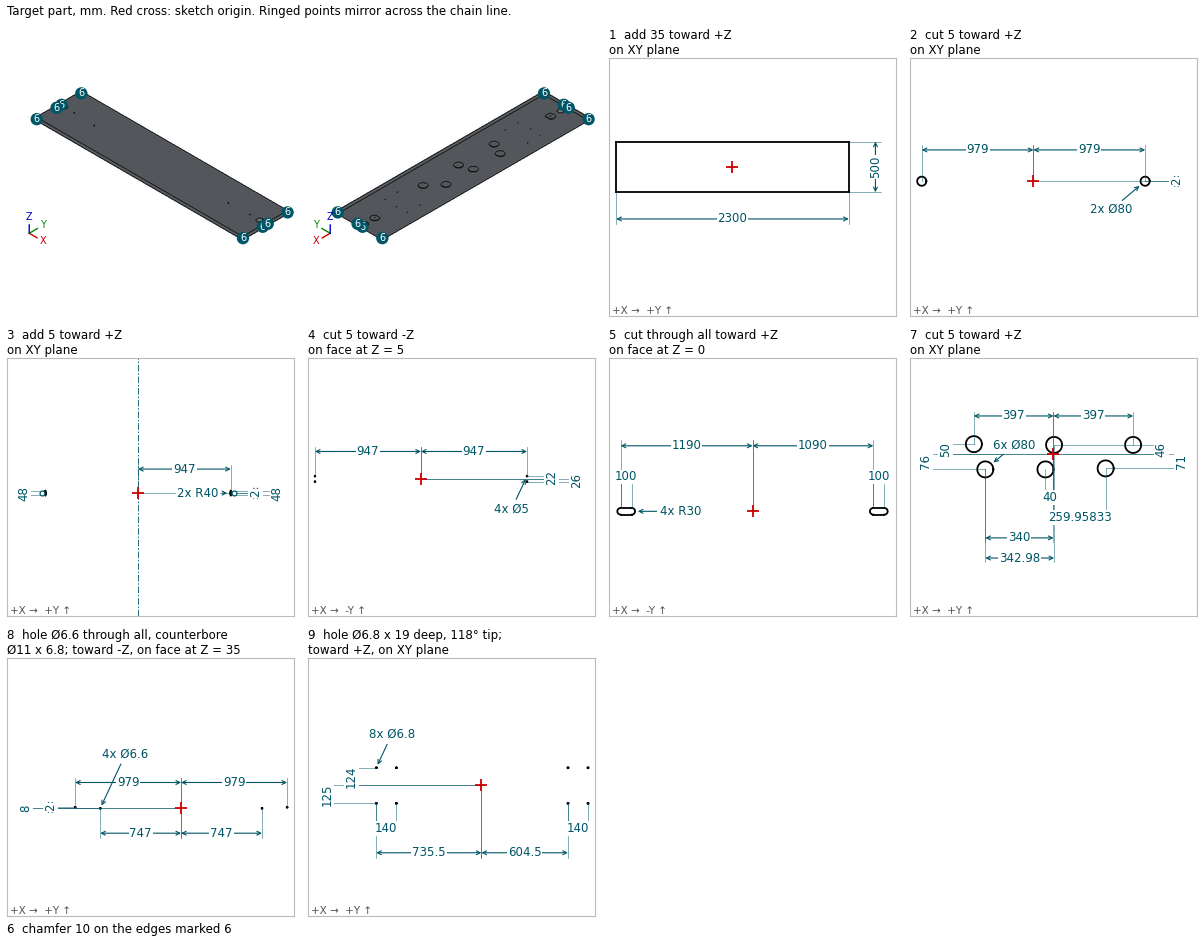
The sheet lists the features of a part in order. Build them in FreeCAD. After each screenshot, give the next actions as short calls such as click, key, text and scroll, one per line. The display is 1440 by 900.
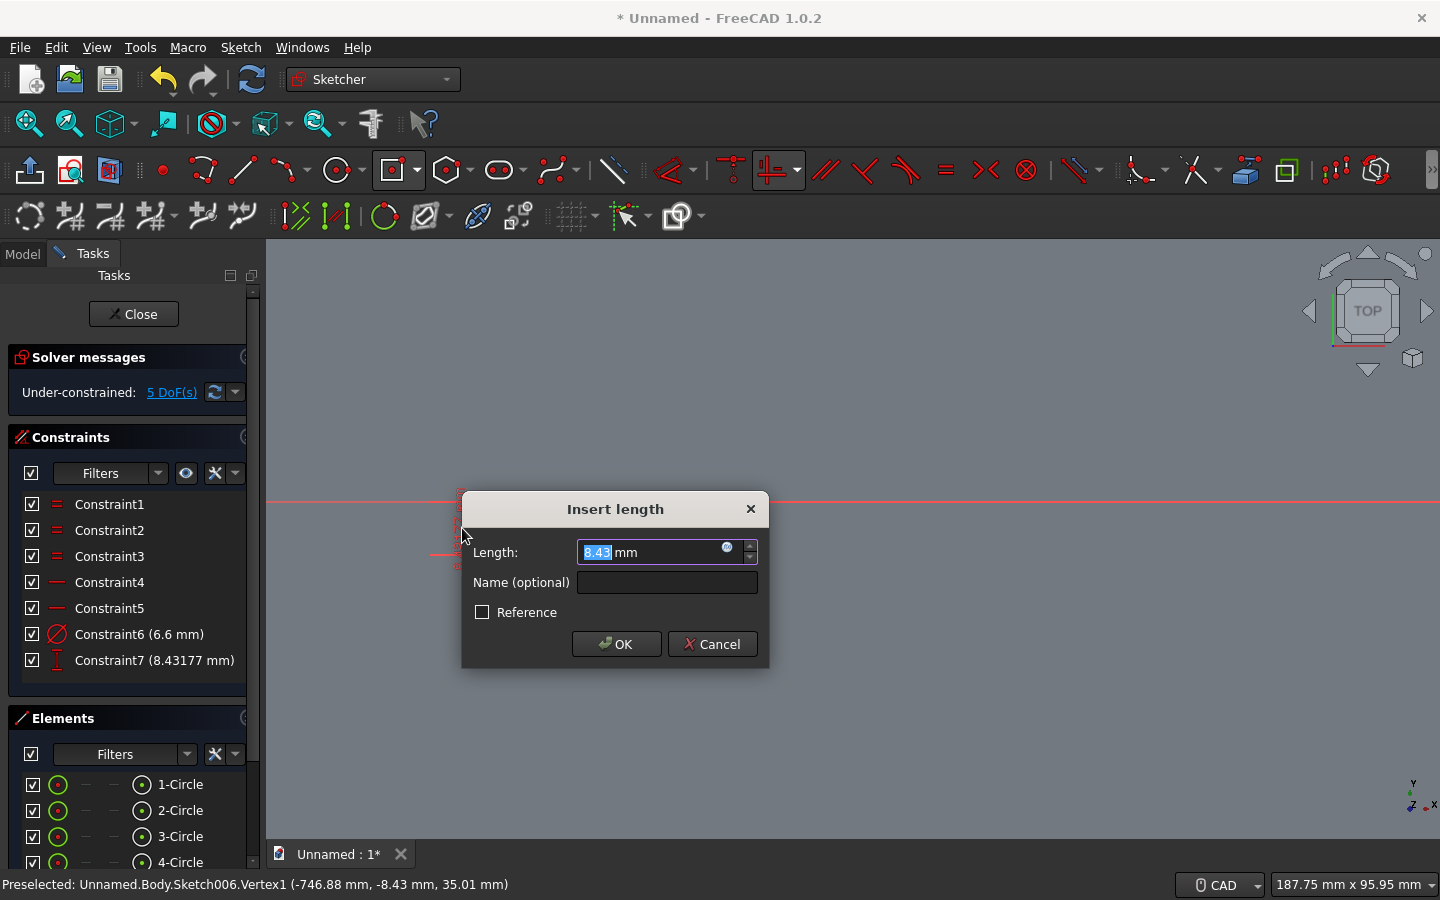
text(8)
key(Return)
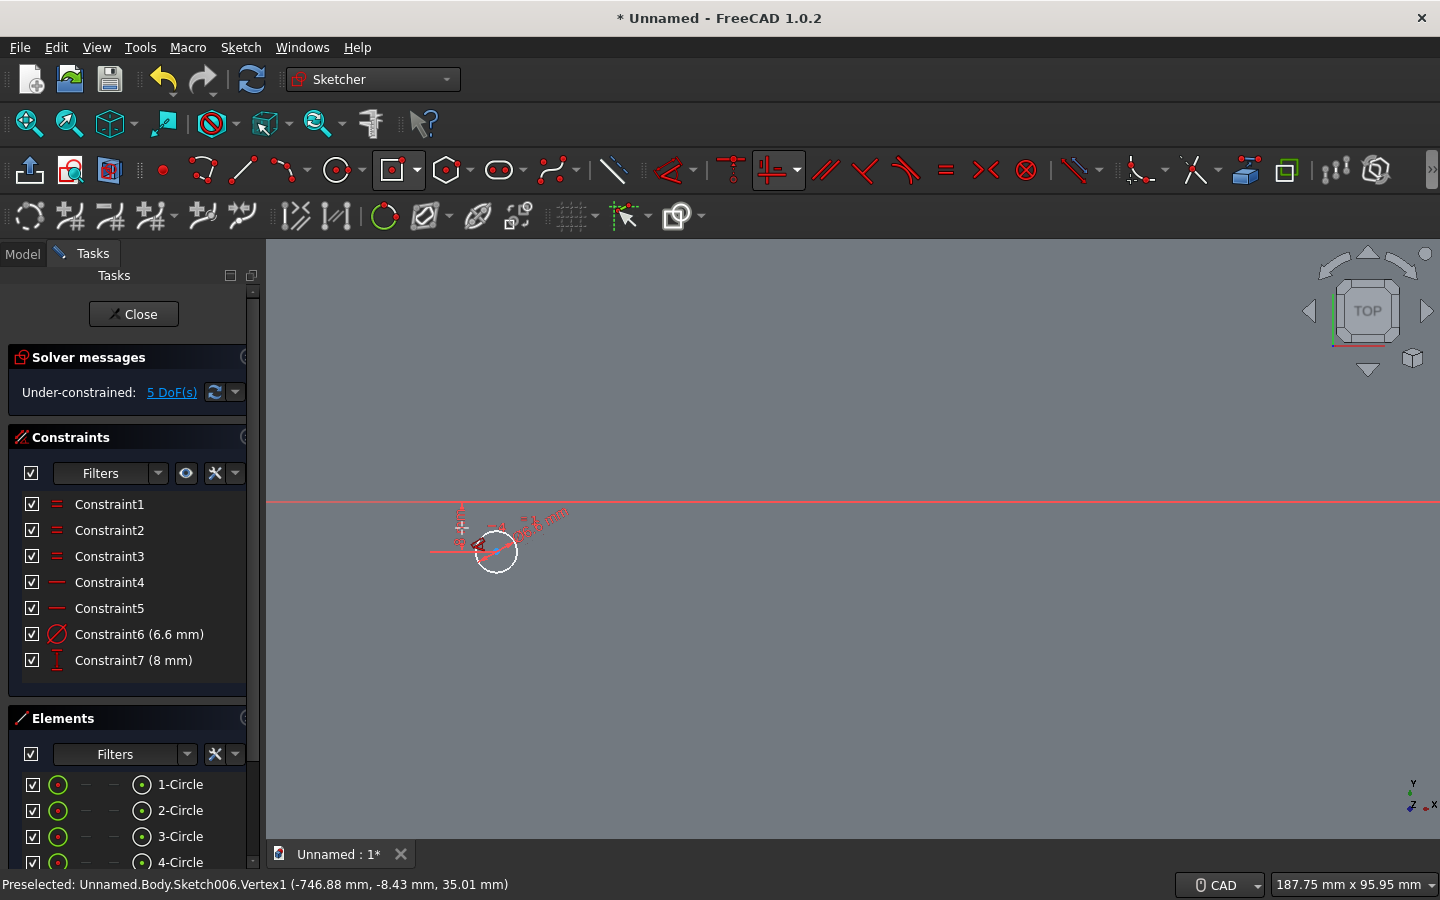
scroll(501, 540, down, 14)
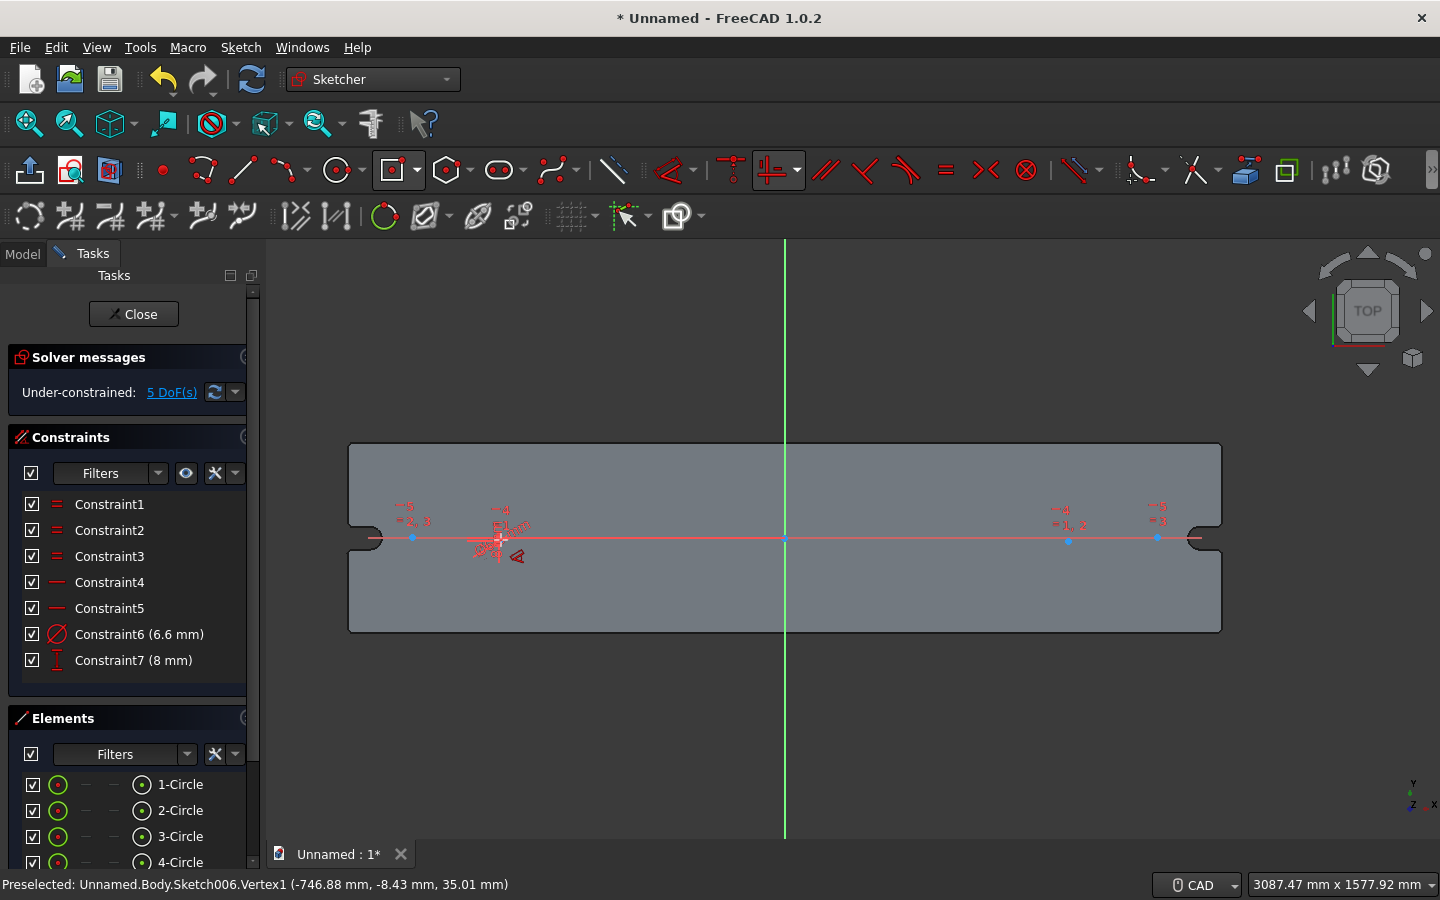
scroll(413, 537, up, 20)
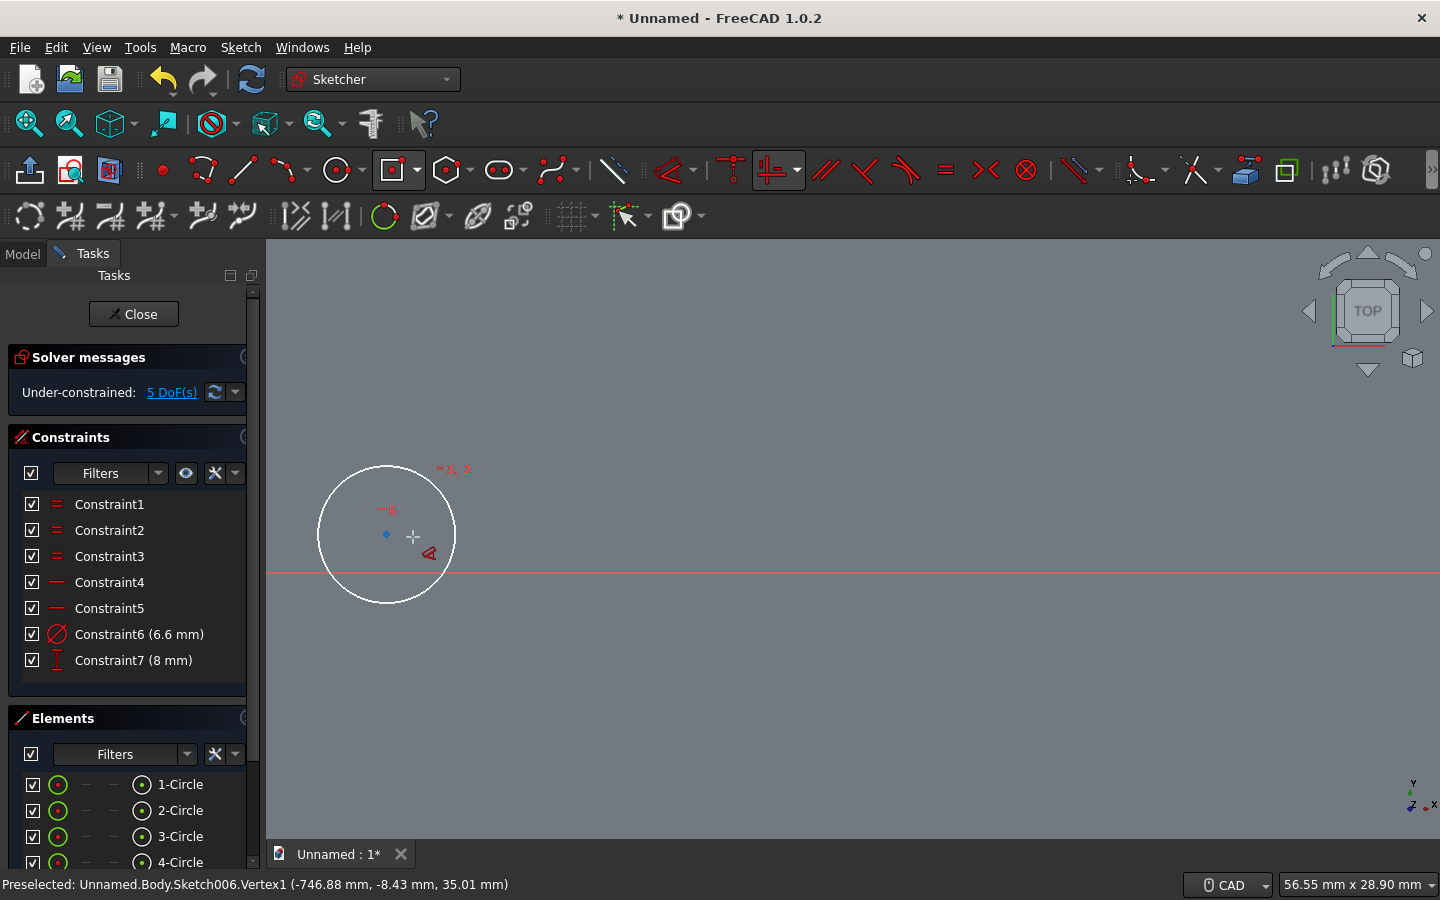
click(387, 535)
click(353, 554)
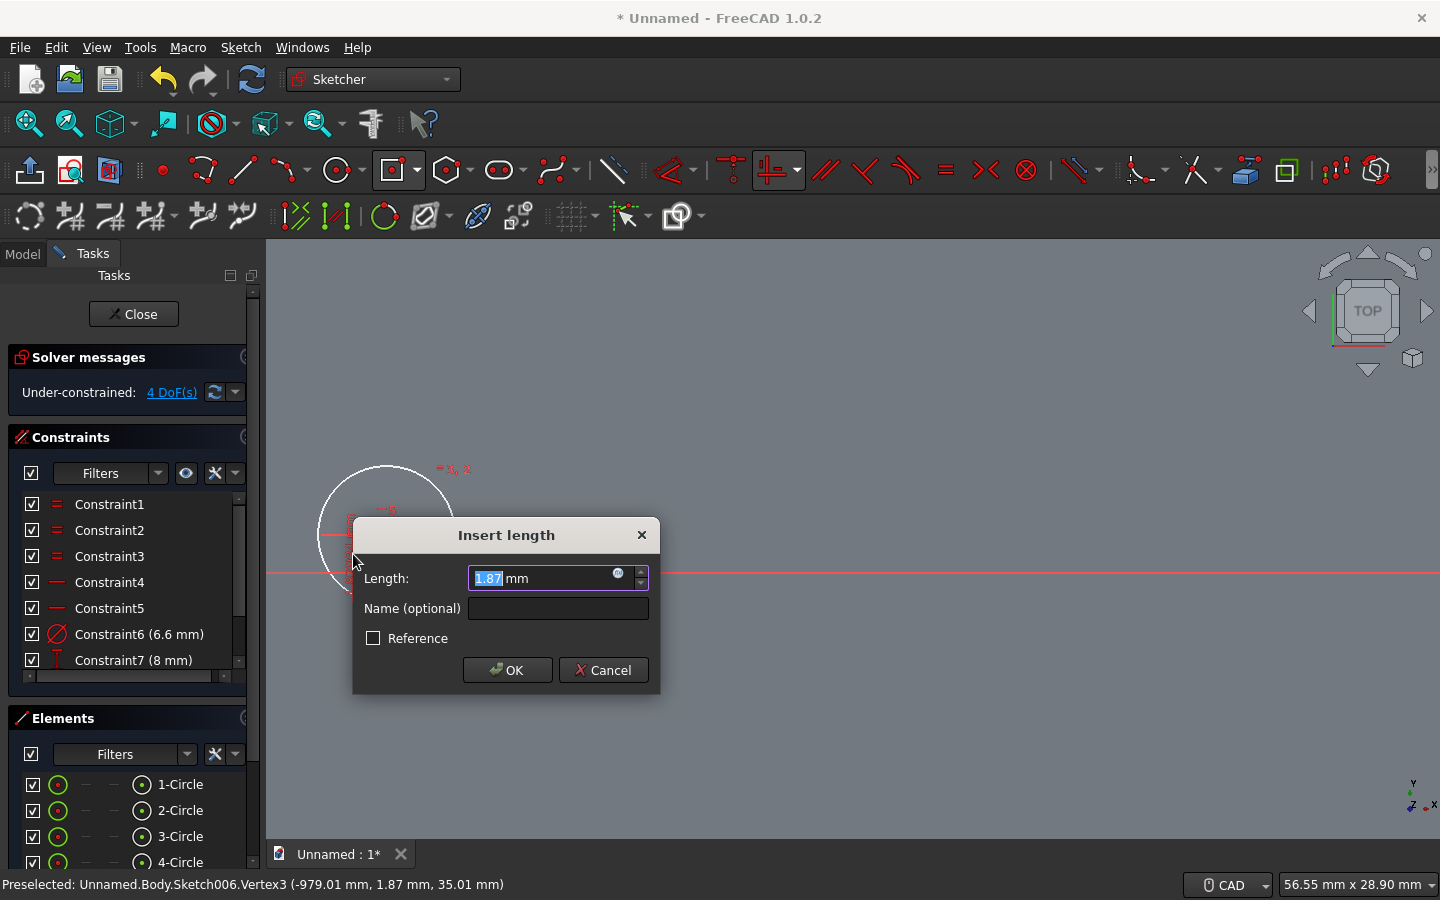
text(2)
key(Return)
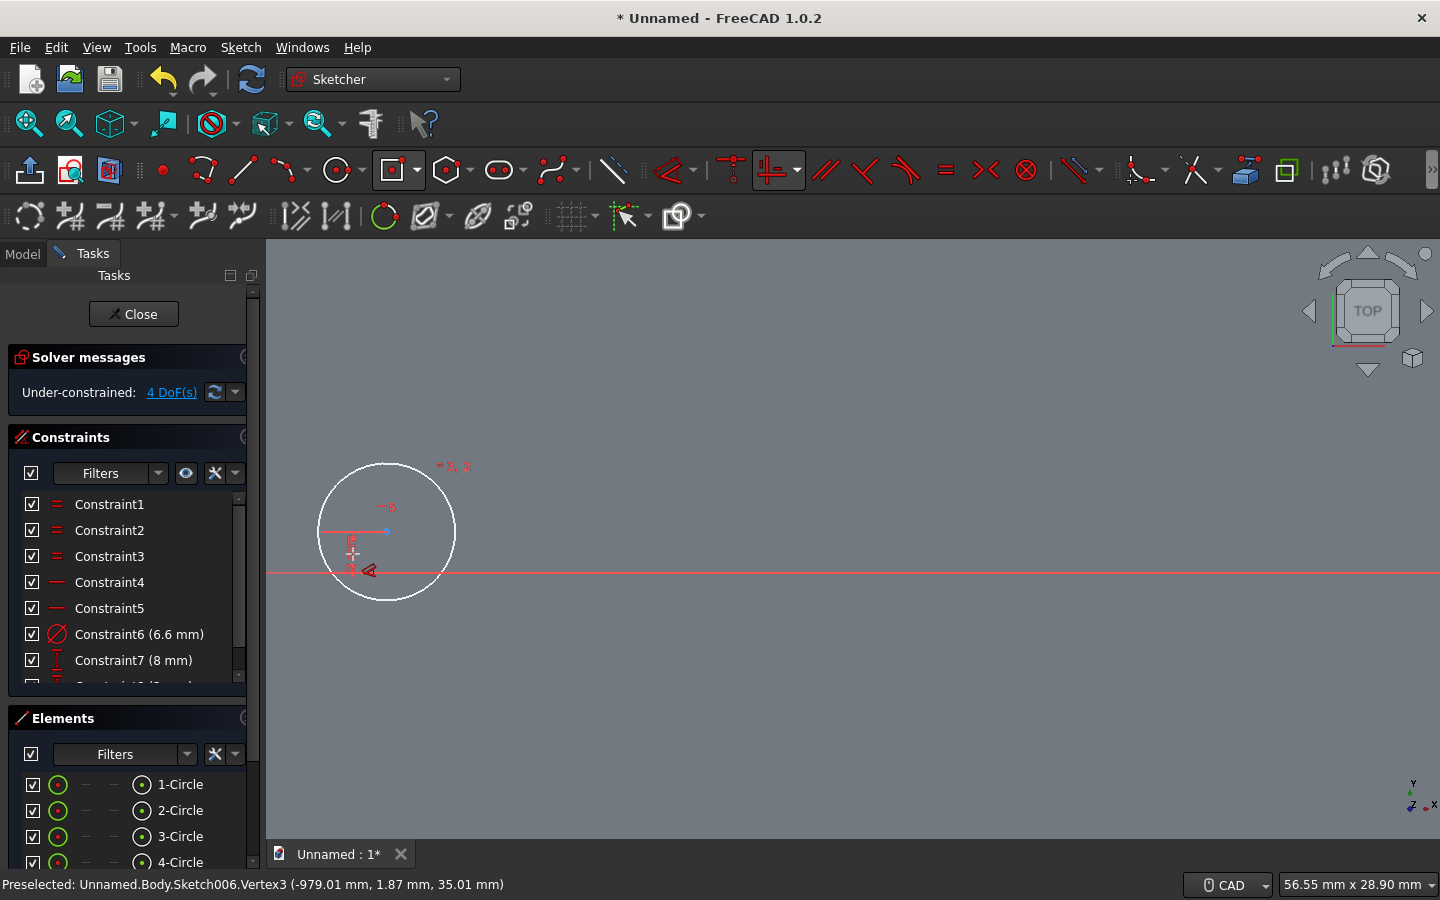
scroll(784, 539, down, 15)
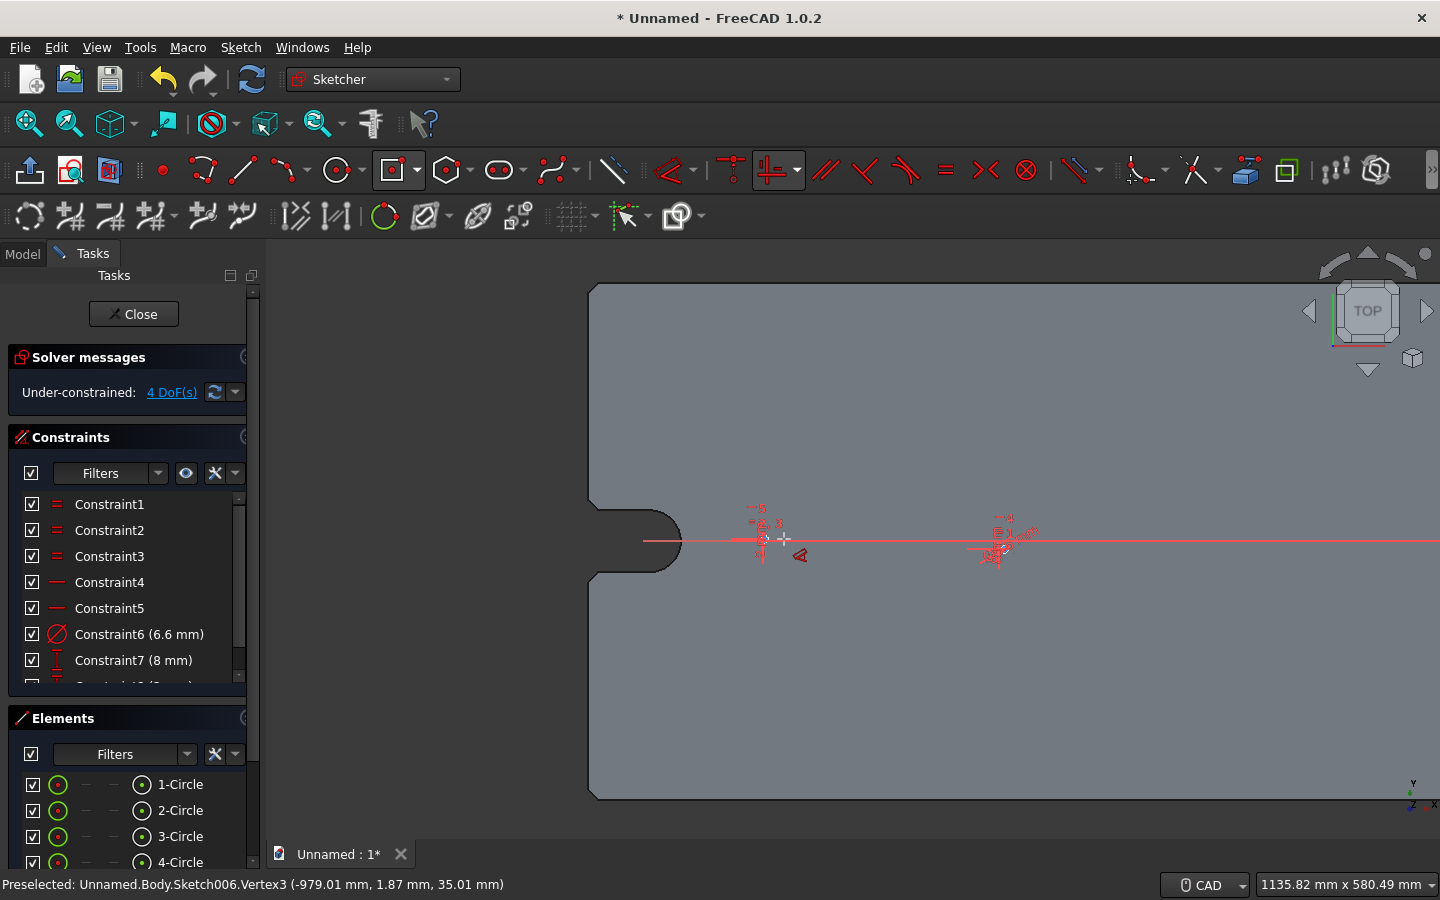
scroll(294, 536, down, 5)